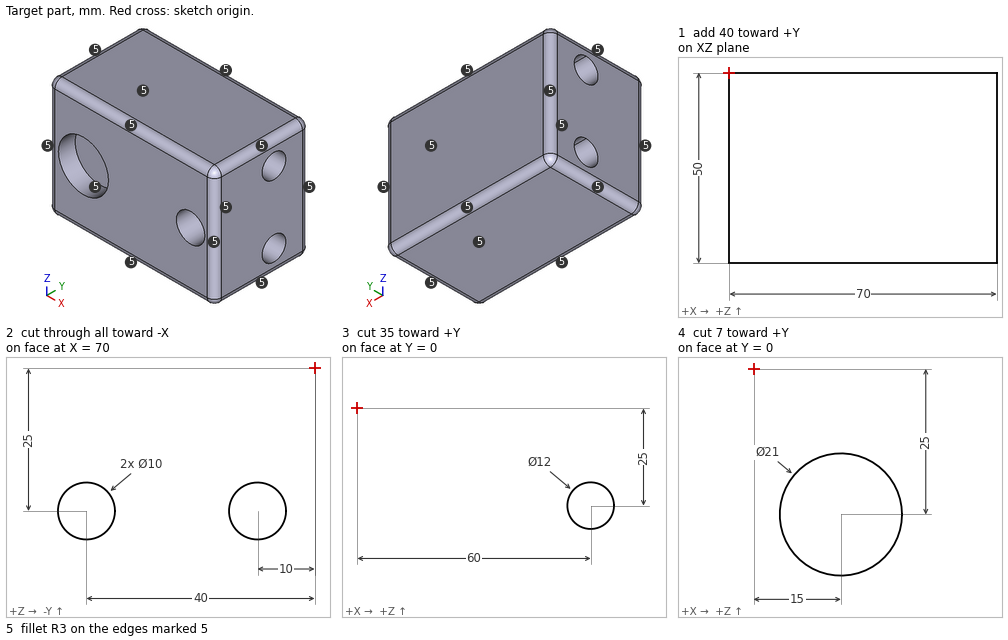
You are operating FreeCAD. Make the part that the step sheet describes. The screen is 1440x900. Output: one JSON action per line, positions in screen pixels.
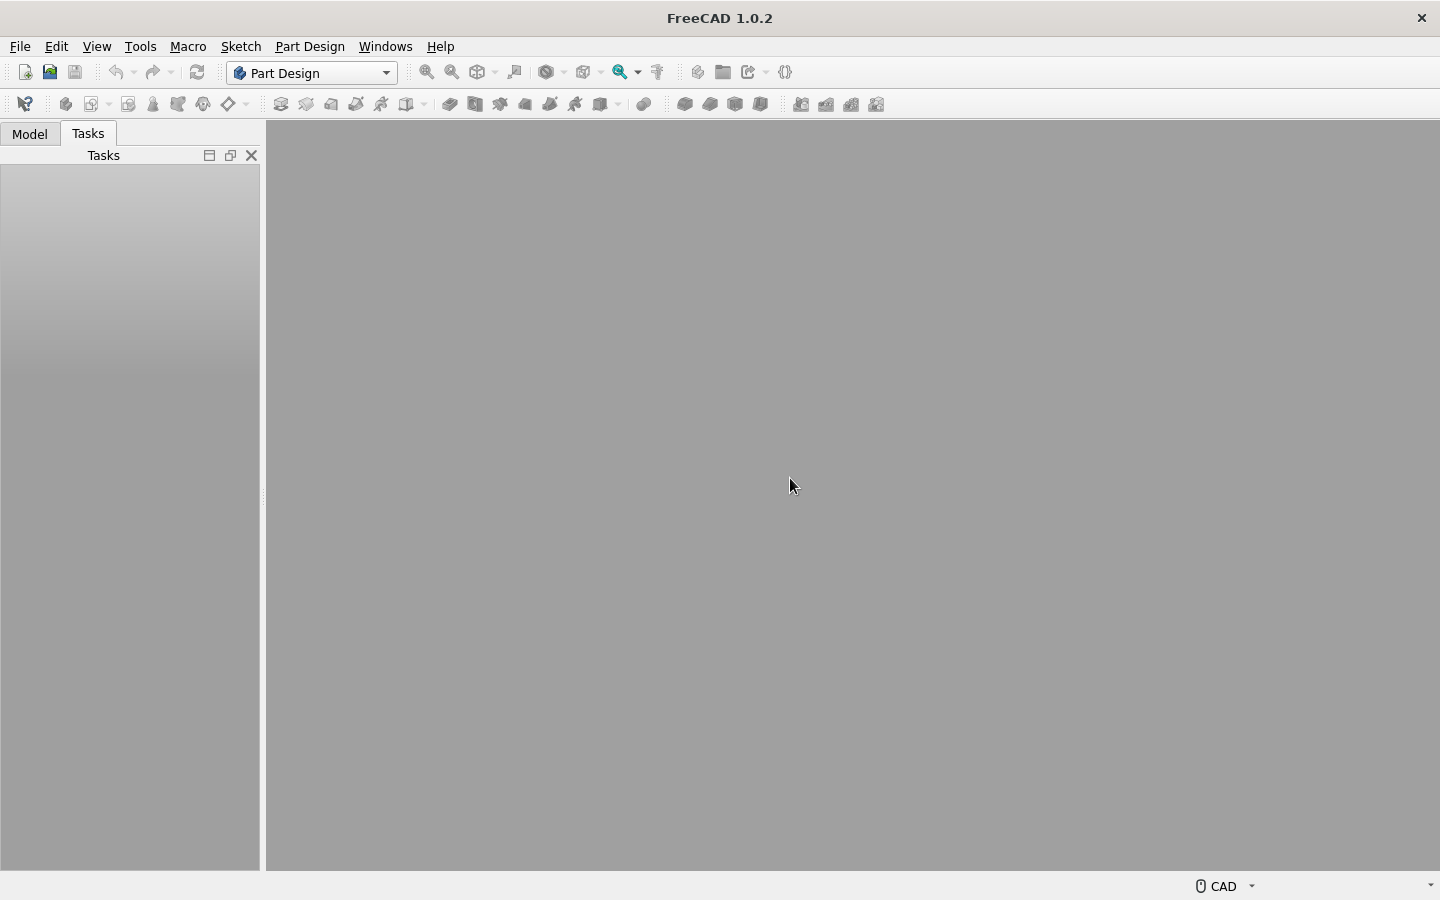
{"action": "key", "text": "ctrl+n"}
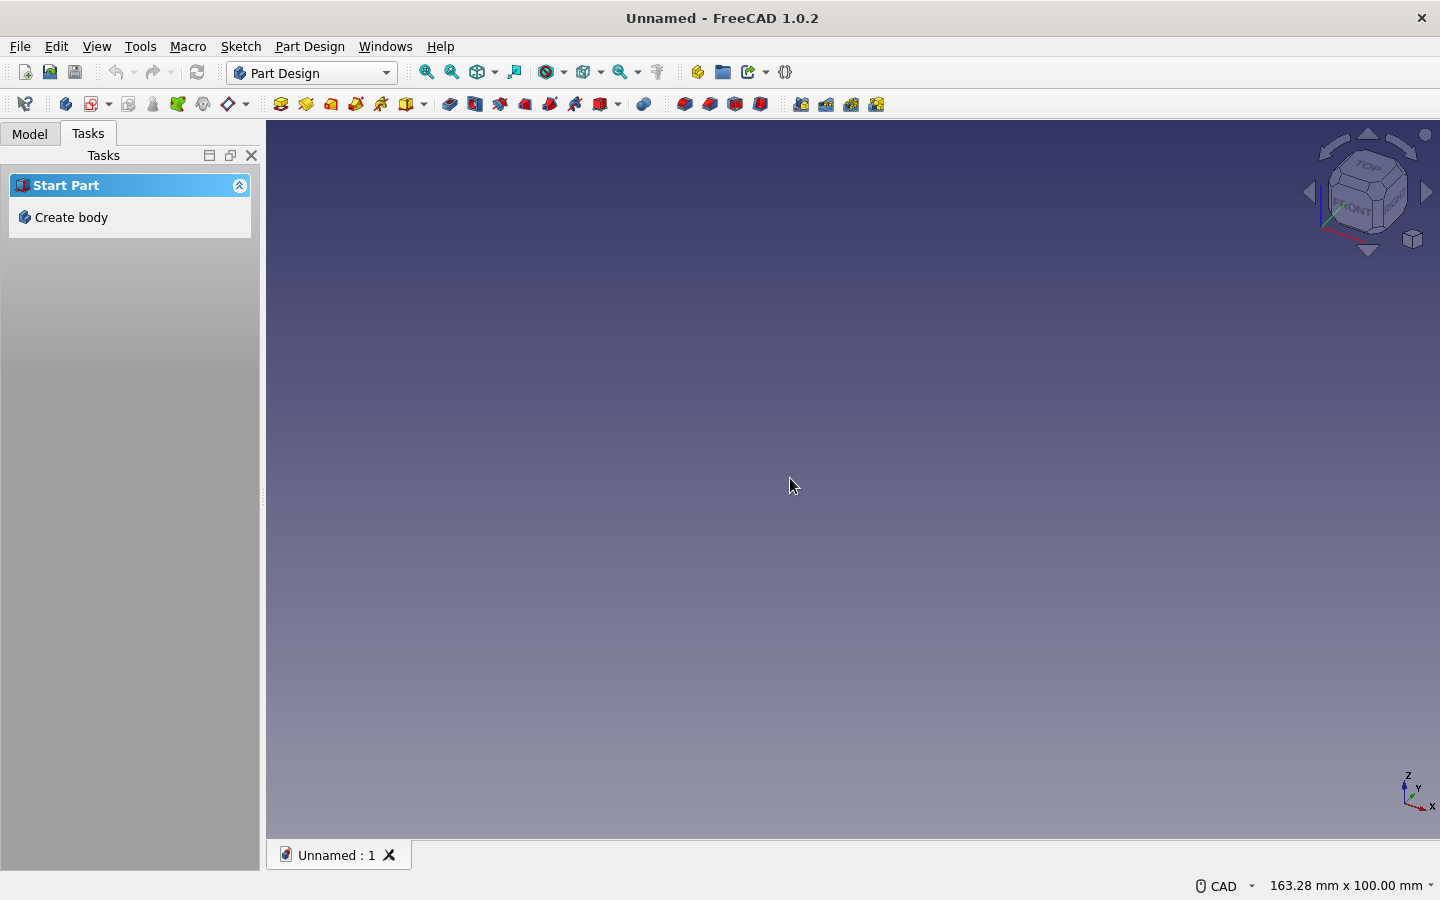
{"action": "left_click", "coordinate": [90, 104]}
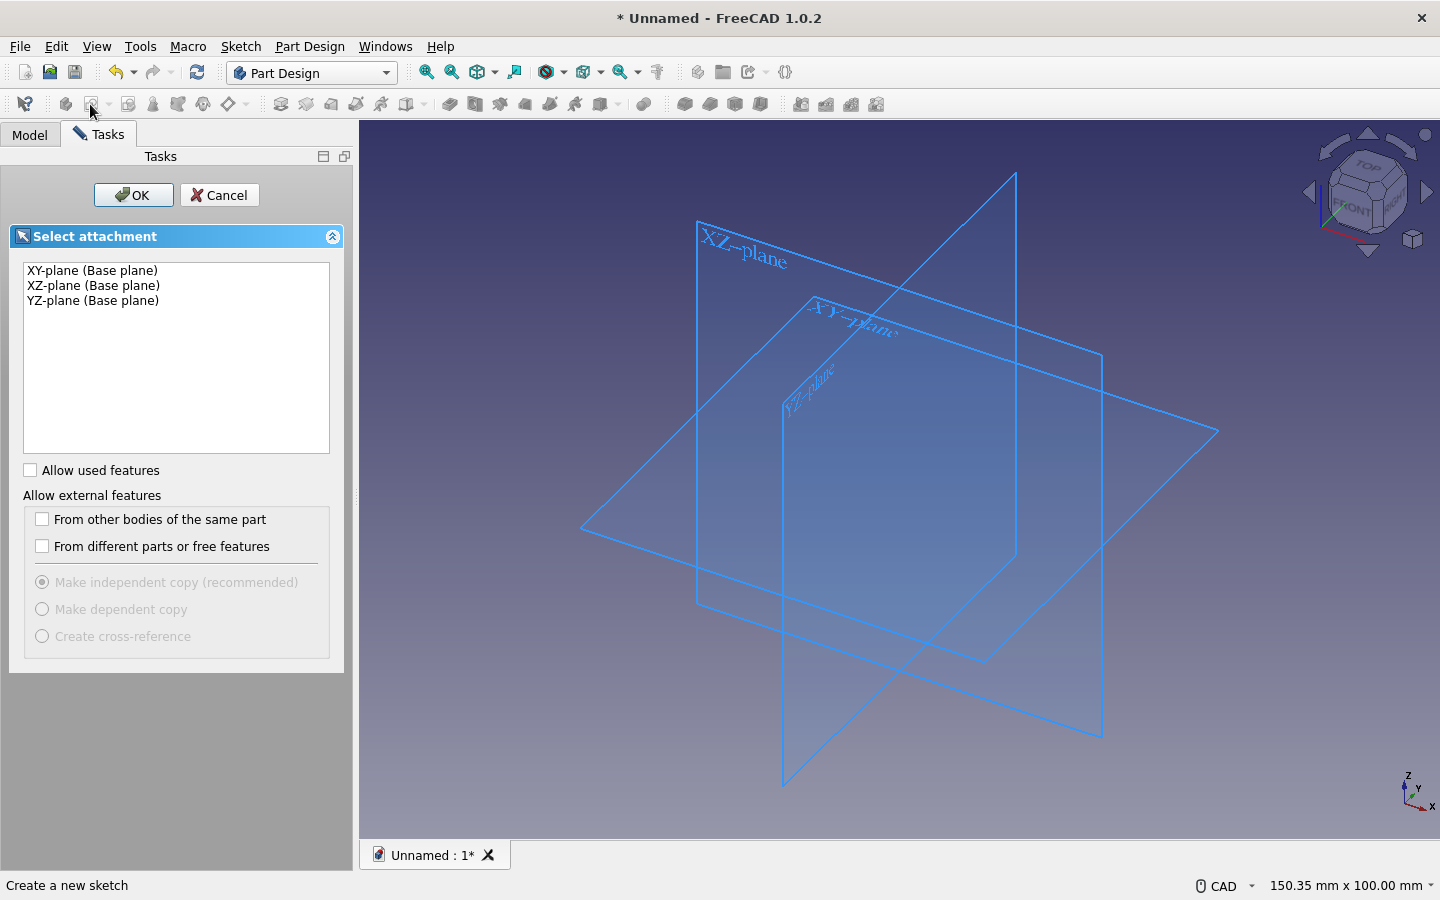
{"action": "left_click", "coordinate": [84, 286]}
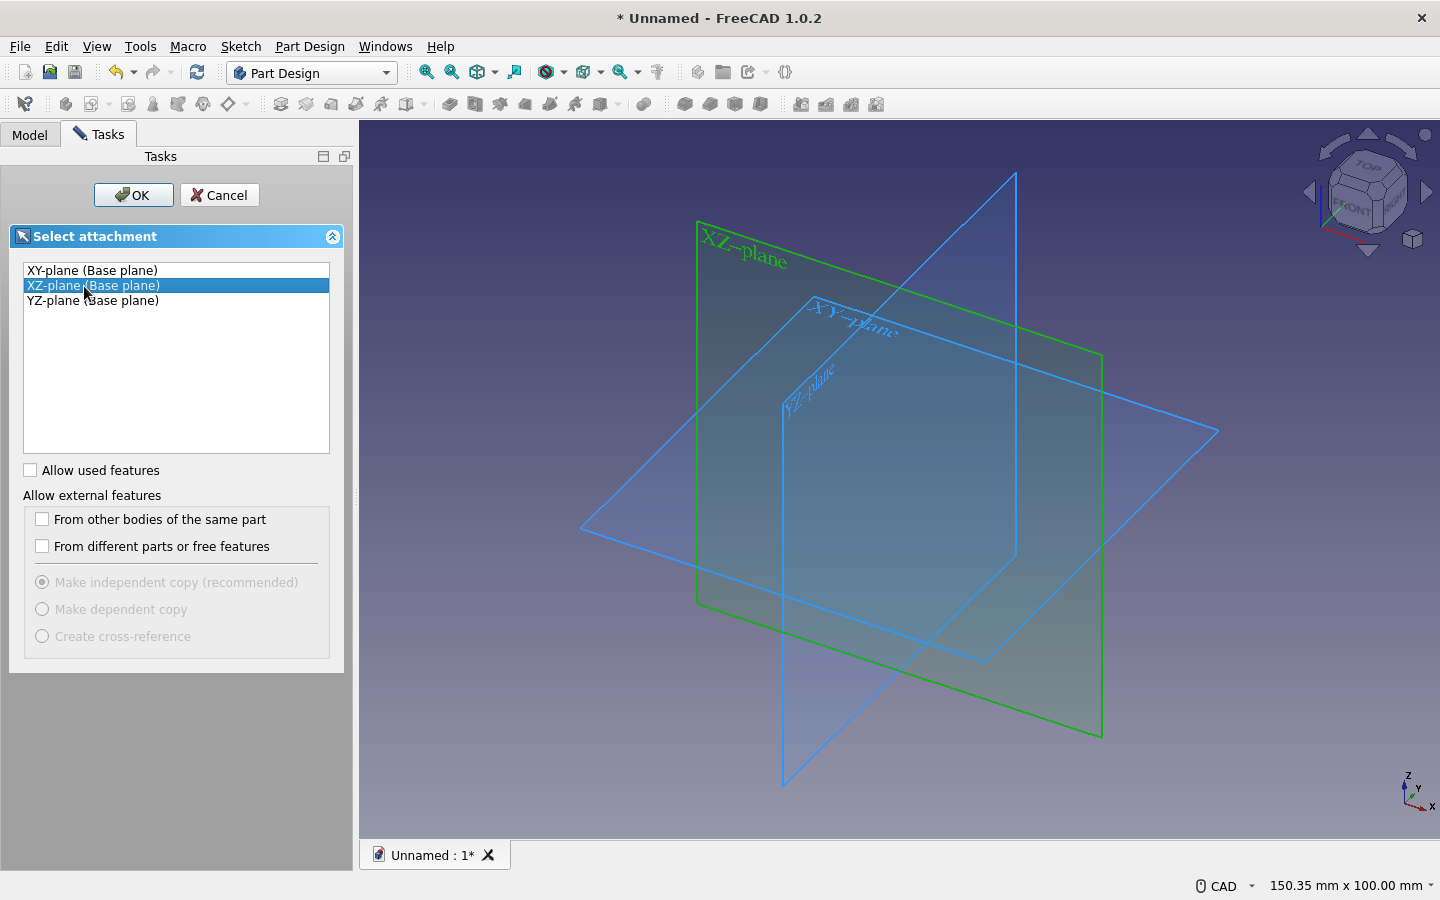
{"action": "left_click", "coordinate": [134, 195]}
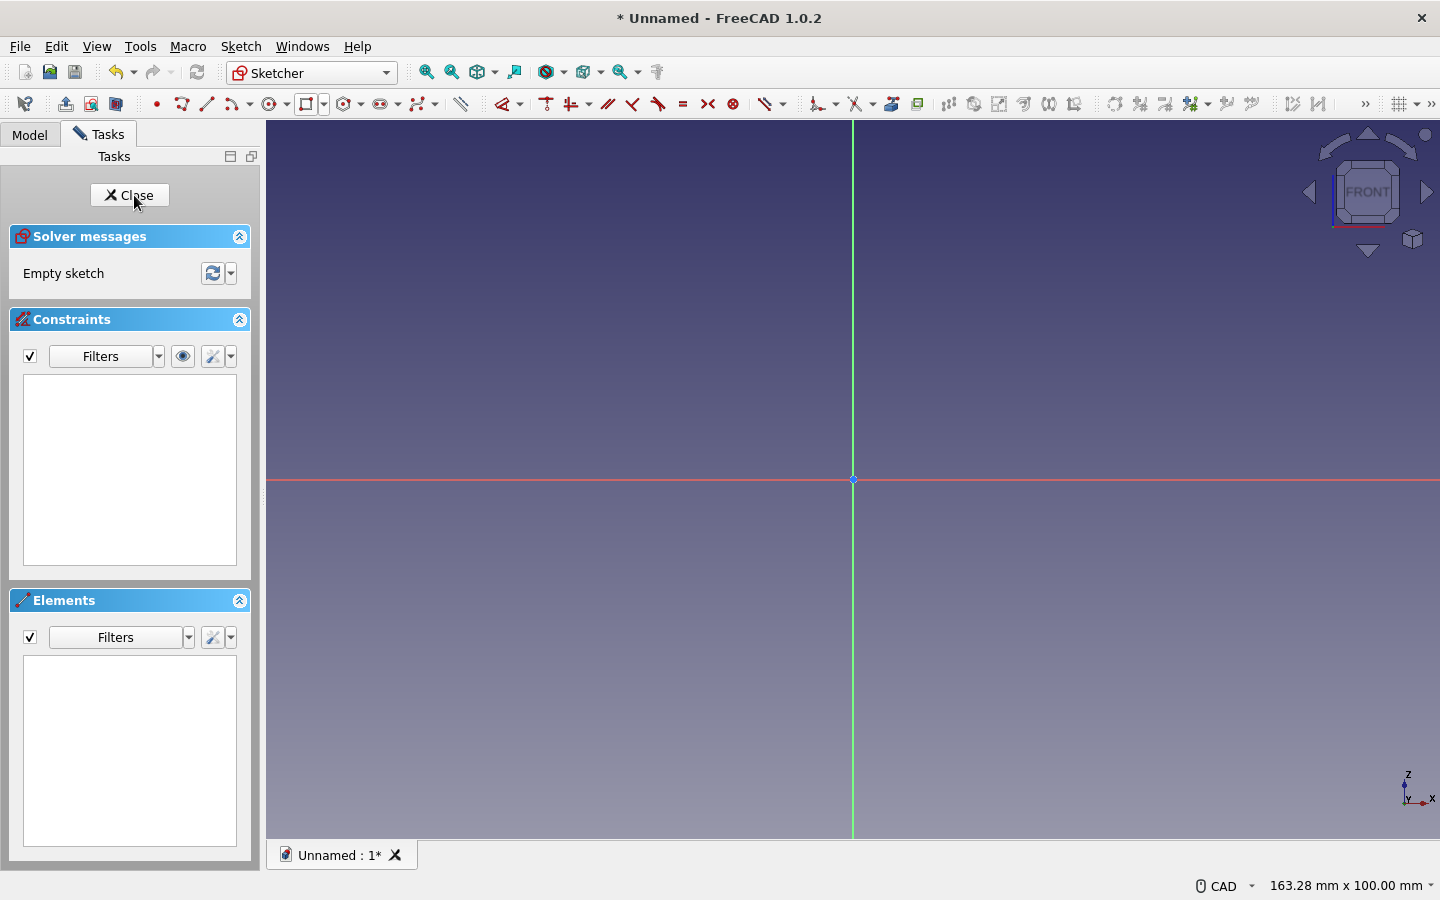
{"action": "scroll", "coordinate": [294, 148], "scroll_direction": "down", "scroll_amount": 1}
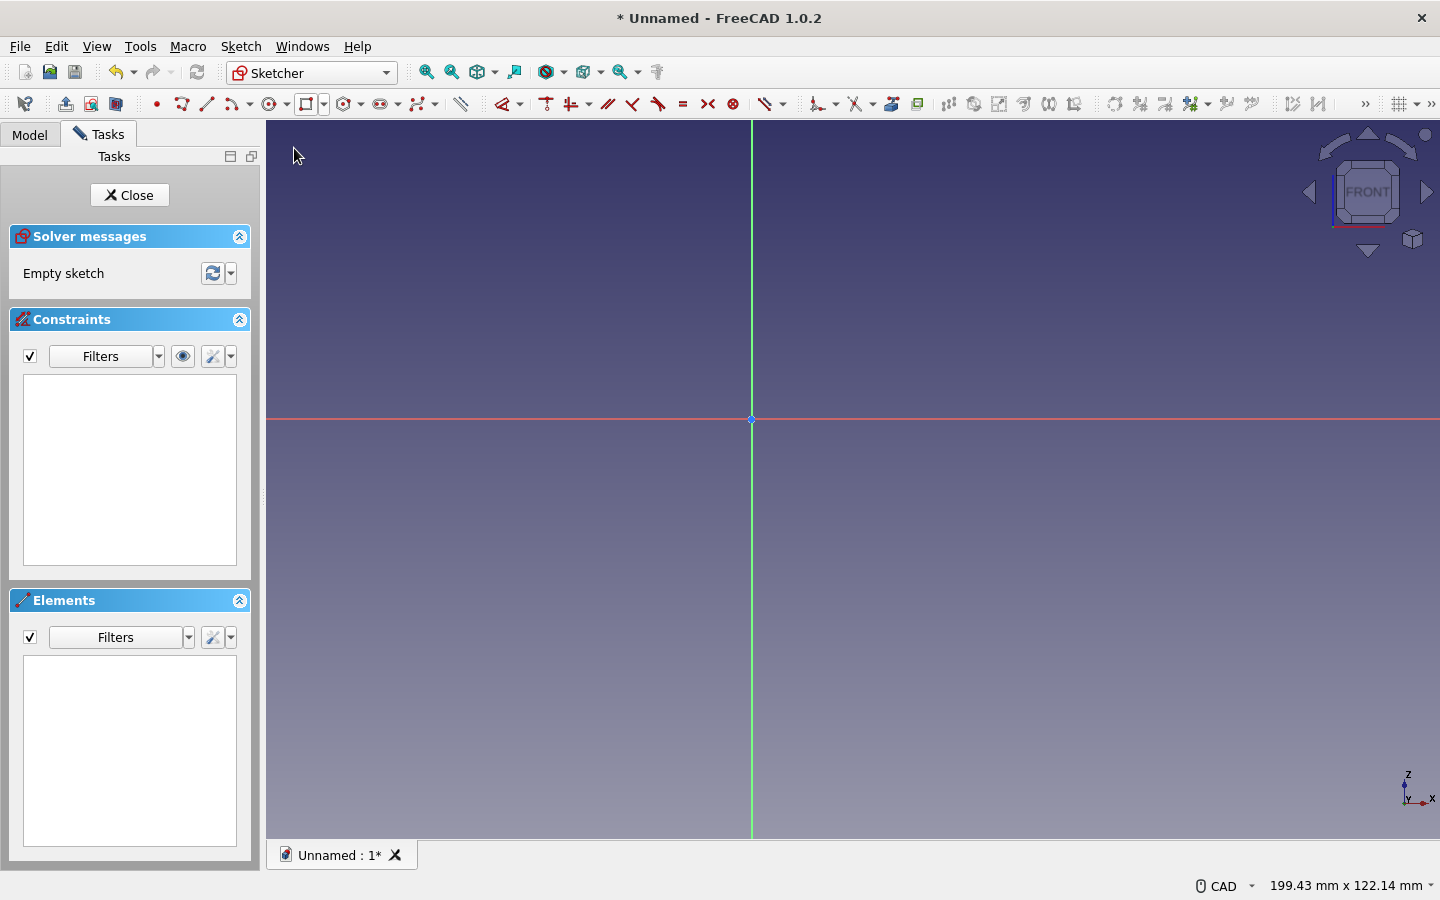
{"action": "scroll", "coordinate": [1275, 744], "scroll_direction": "up", "scroll_amount": 2}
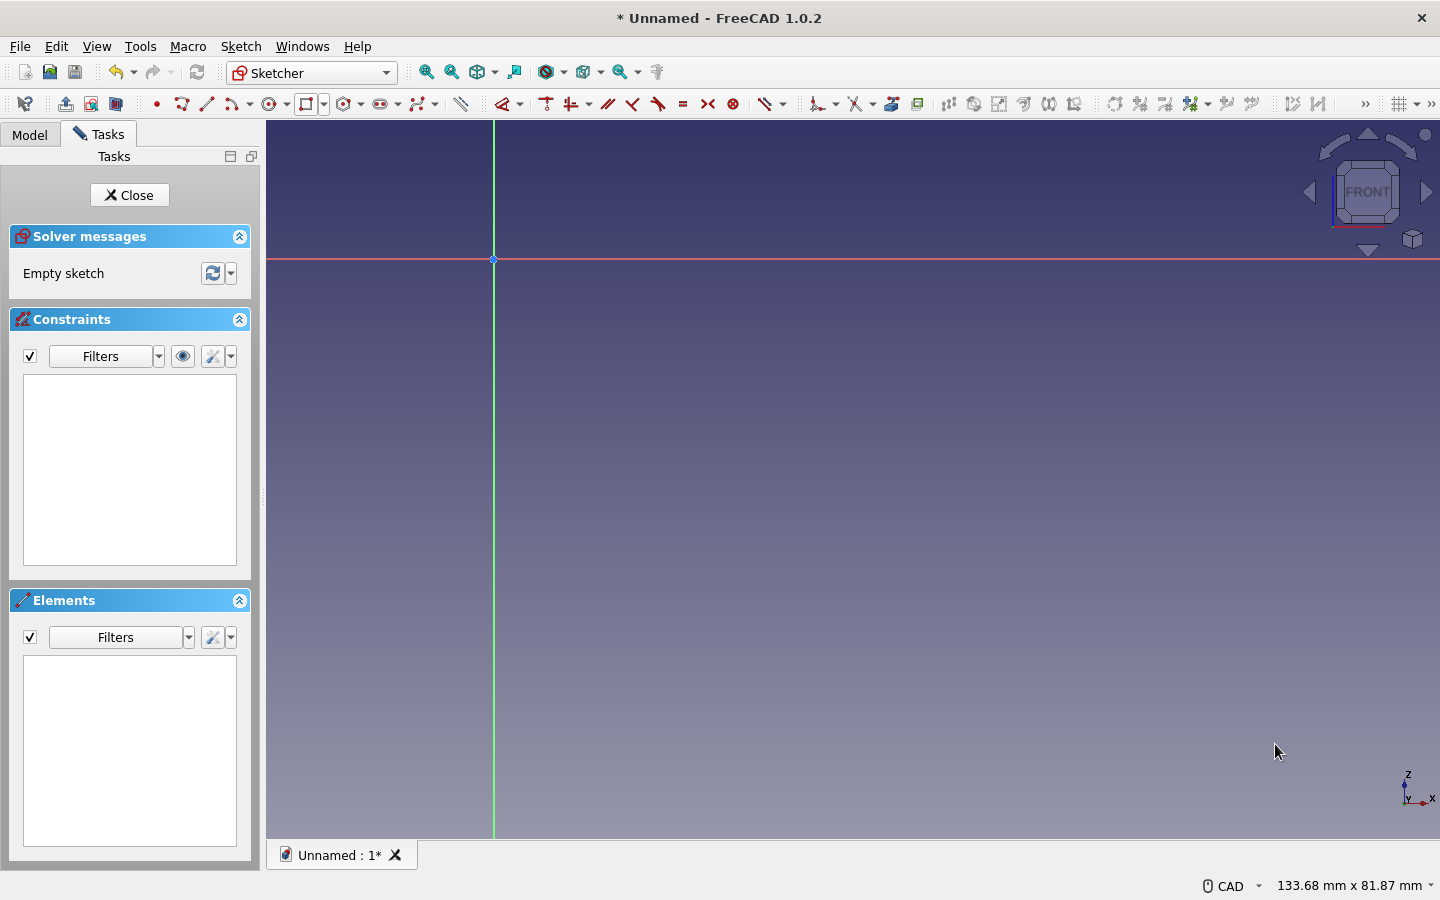
{"action": "key", "text": "g r"}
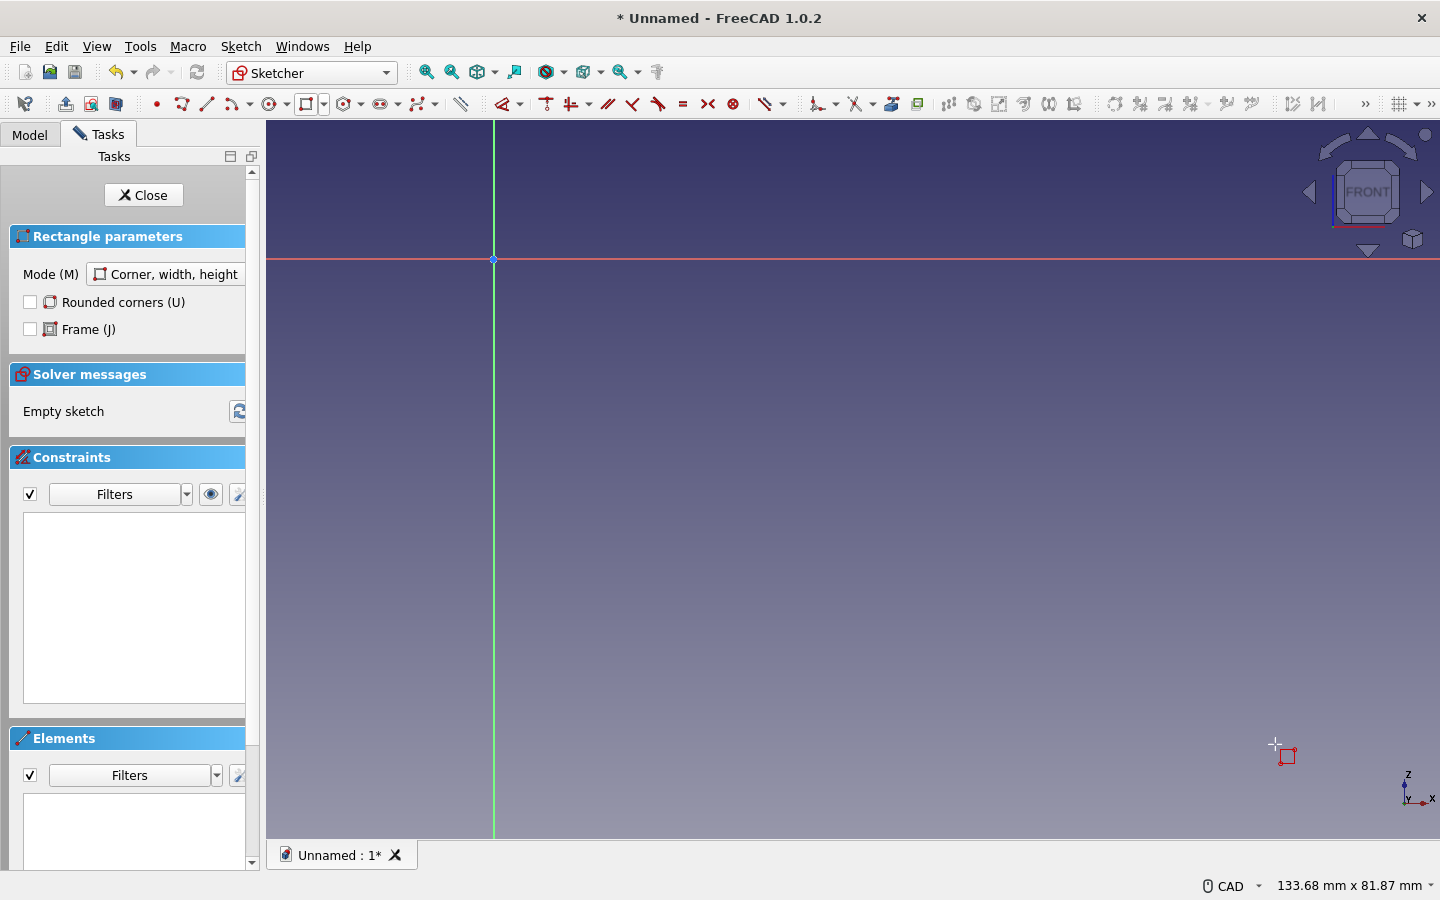
{"action": "left_click", "coordinate": [494, 259]}
{"action": "left_click", "coordinate": [1109, 698]}
{"action": "key", "text": "Escape"}